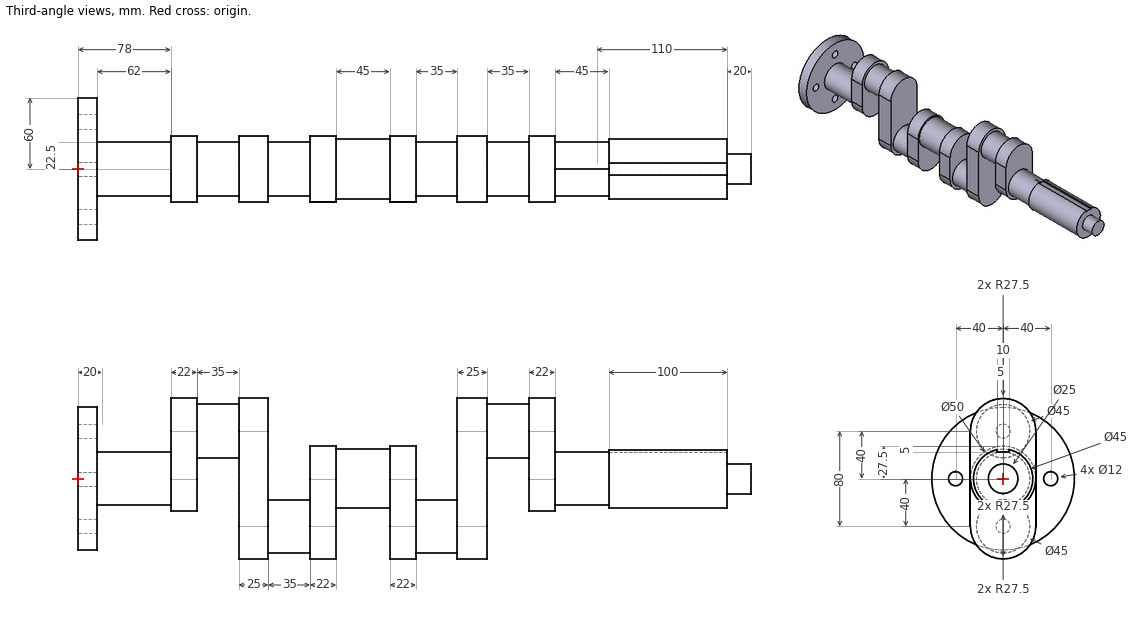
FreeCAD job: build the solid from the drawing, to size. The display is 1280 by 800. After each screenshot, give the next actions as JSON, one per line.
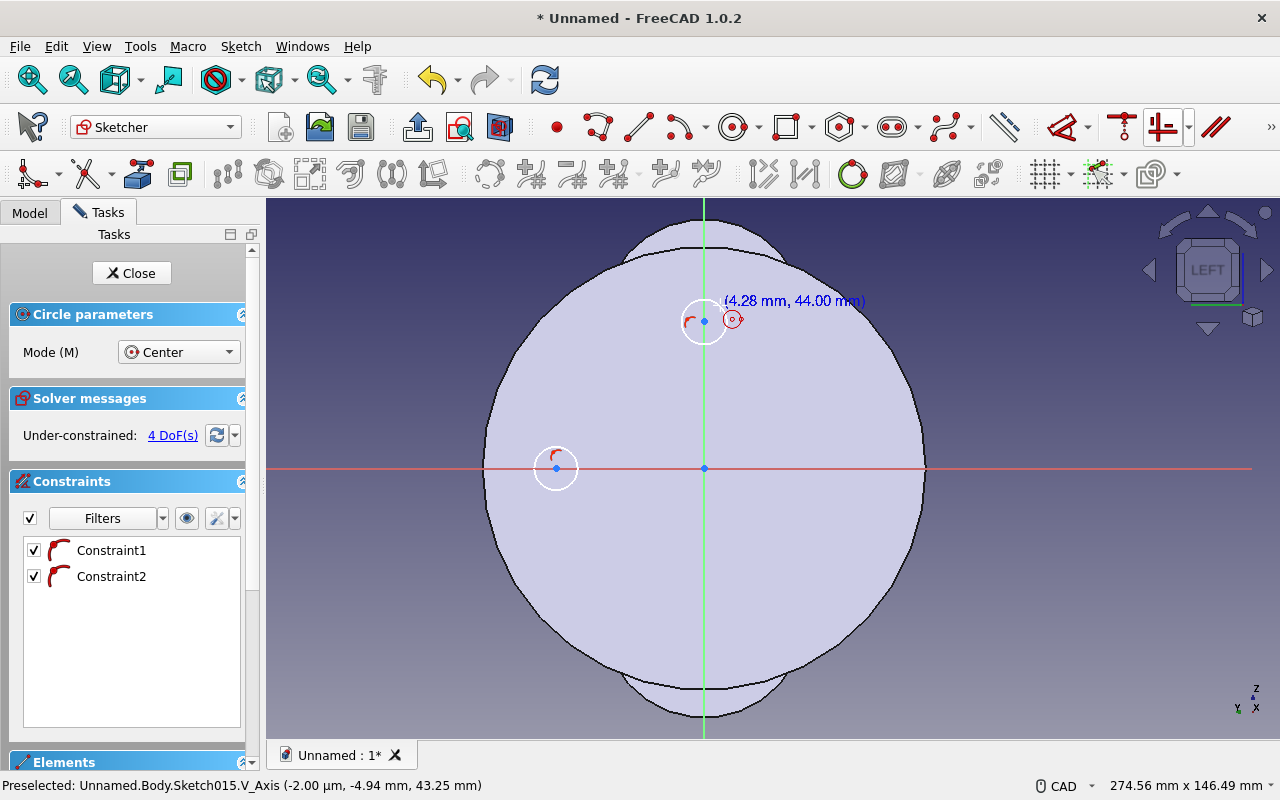
{"action": "left_click", "coordinate": [852, 468]}
{"action": "left_click", "coordinate": [868, 453]}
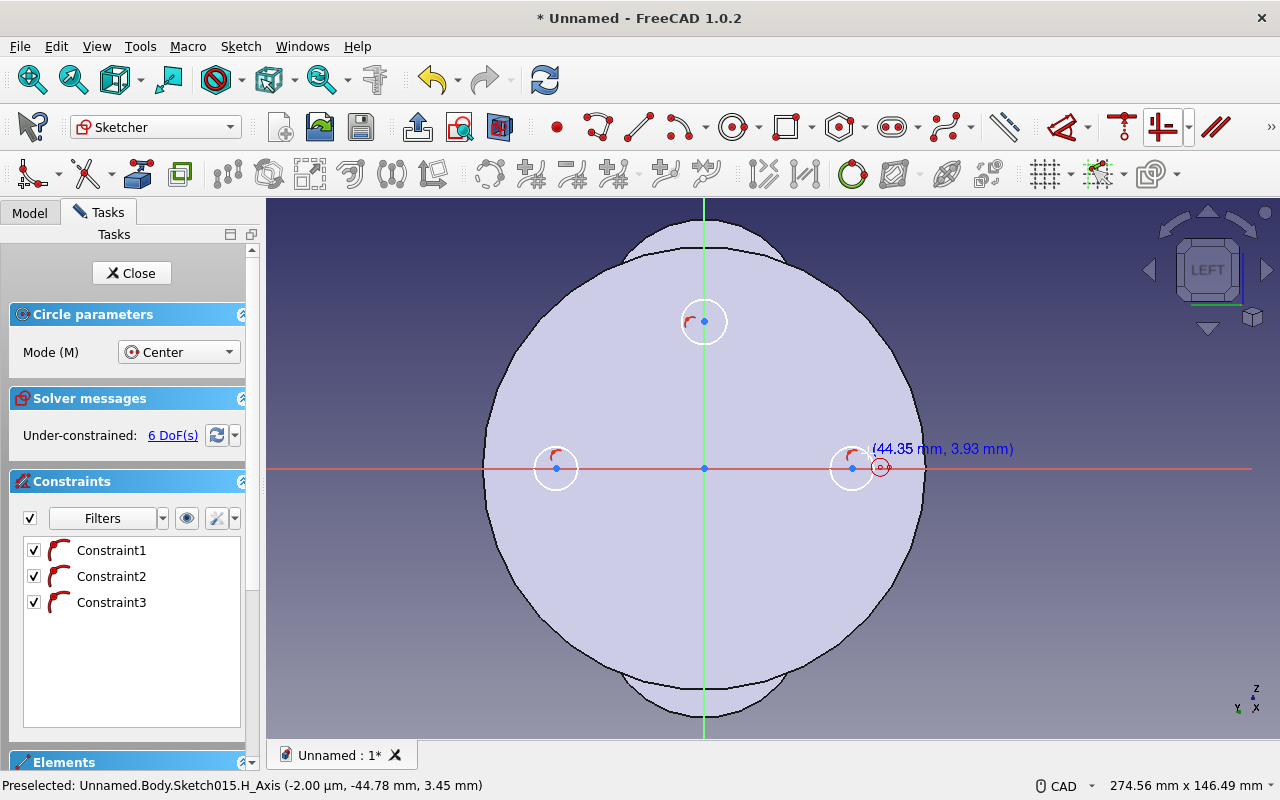
{"action": "left_click", "coordinate": [704, 616]}
{"action": "left_click", "coordinate": [720, 601]}
{"action": "key", "text": "Escape"}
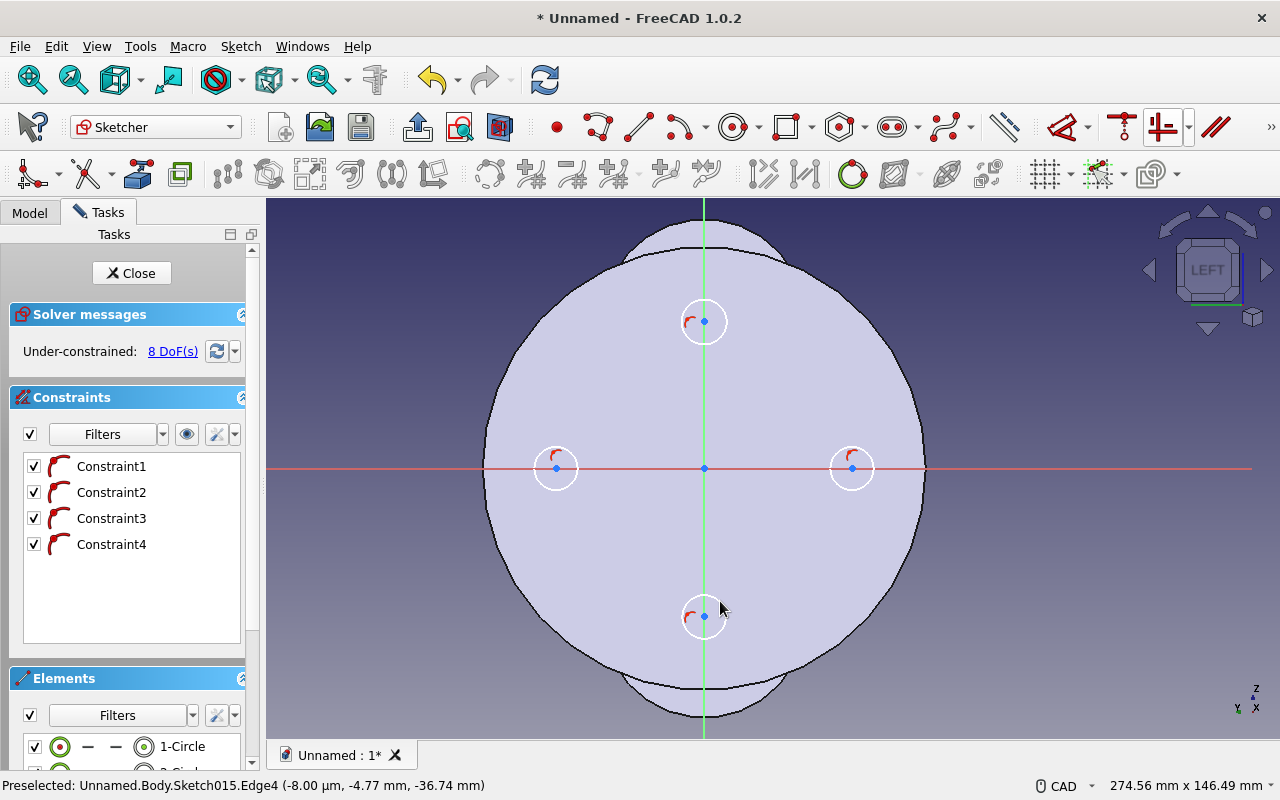
{"action": "left_click", "coordinate": [571, 453]}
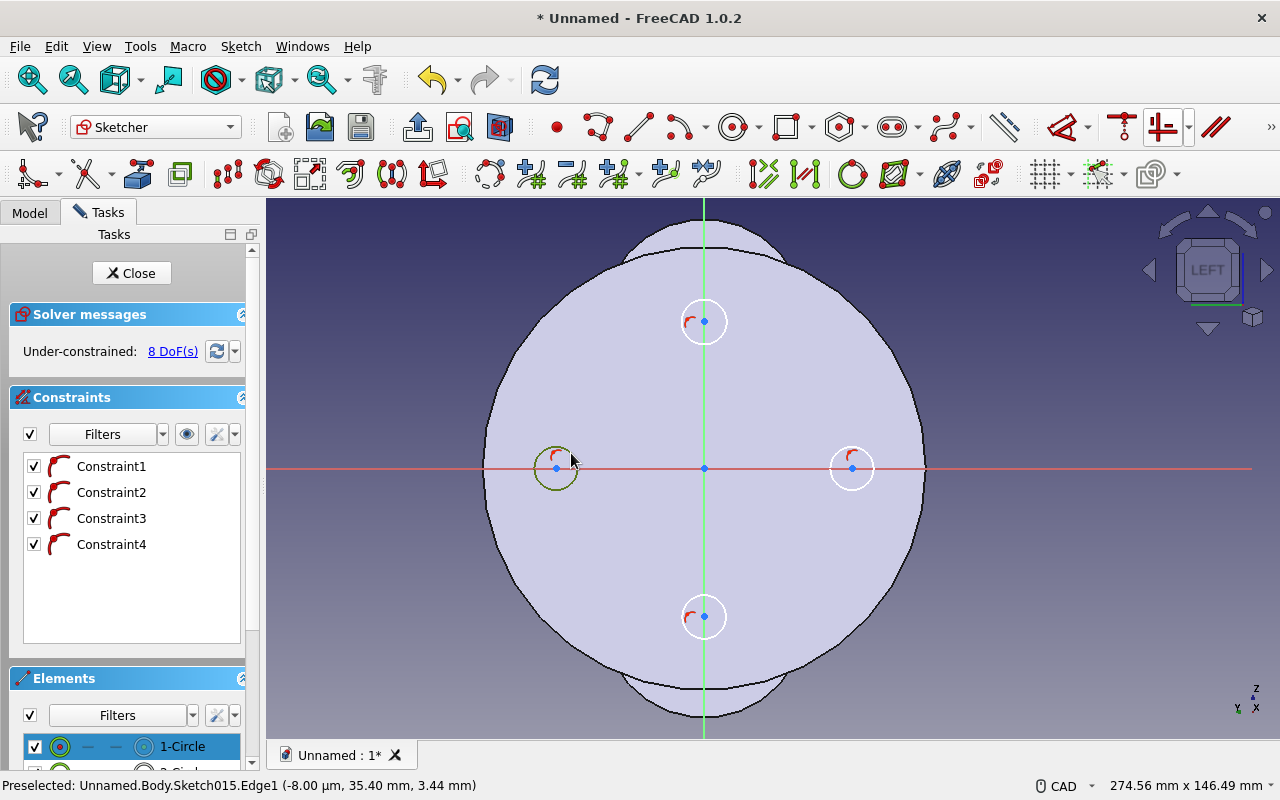
{"action": "left_click", "coordinate": [720, 306]}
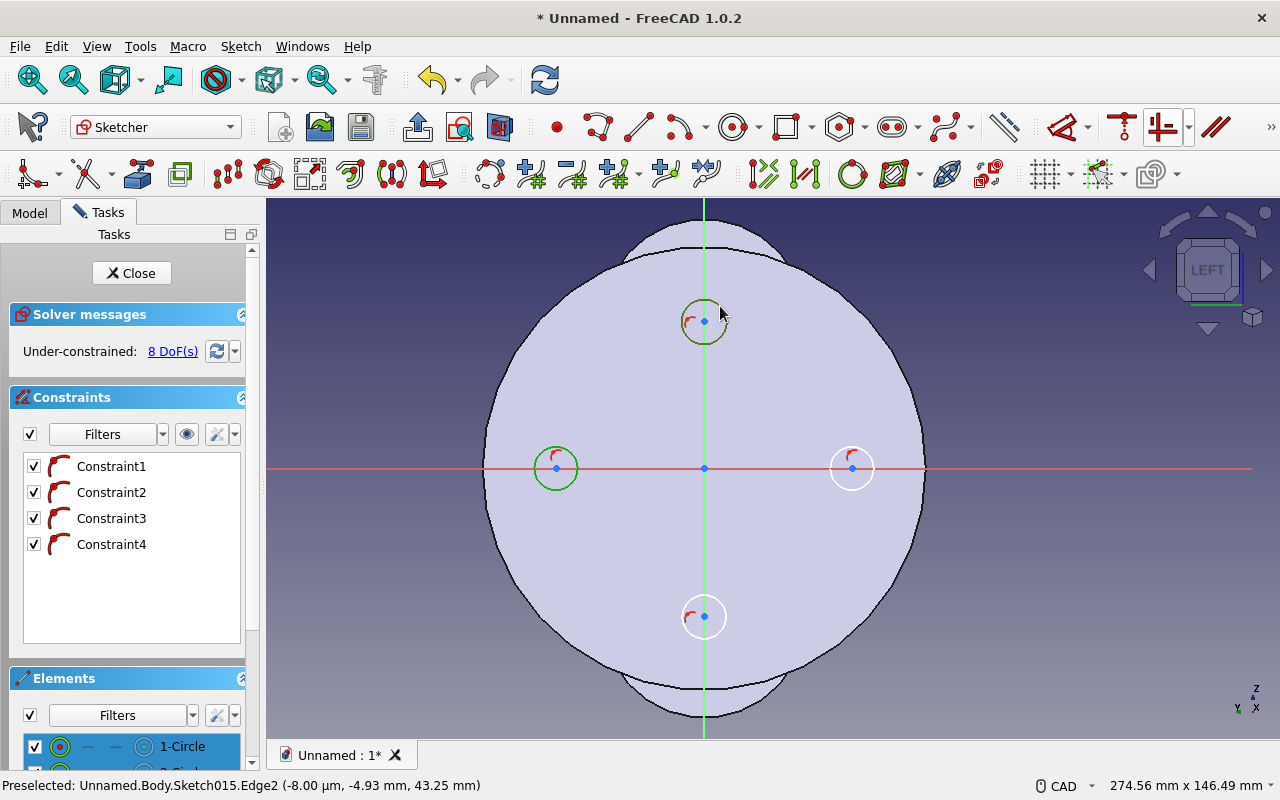
{"action": "left_click", "coordinate": [867, 453]}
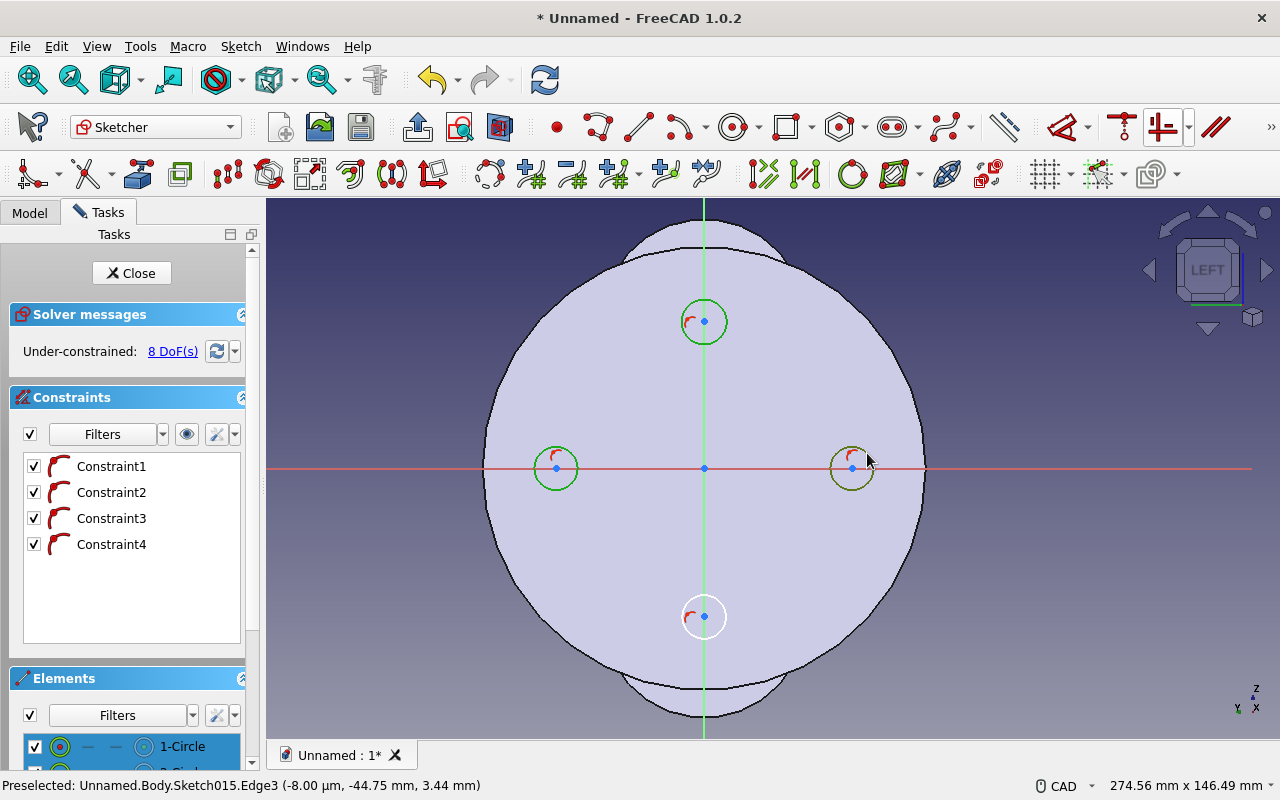
{"action": "left_click", "coordinate": [720, 602]}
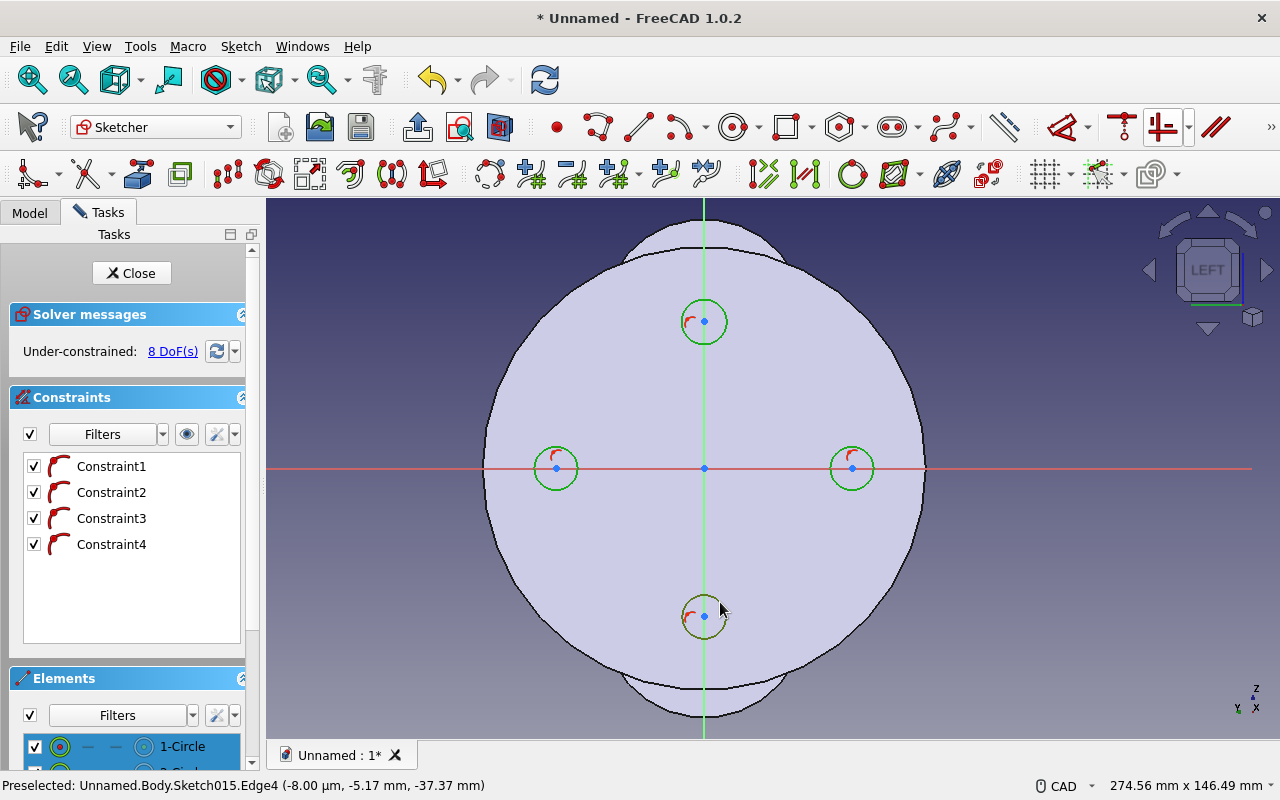
{"action": "key", "text": "e"}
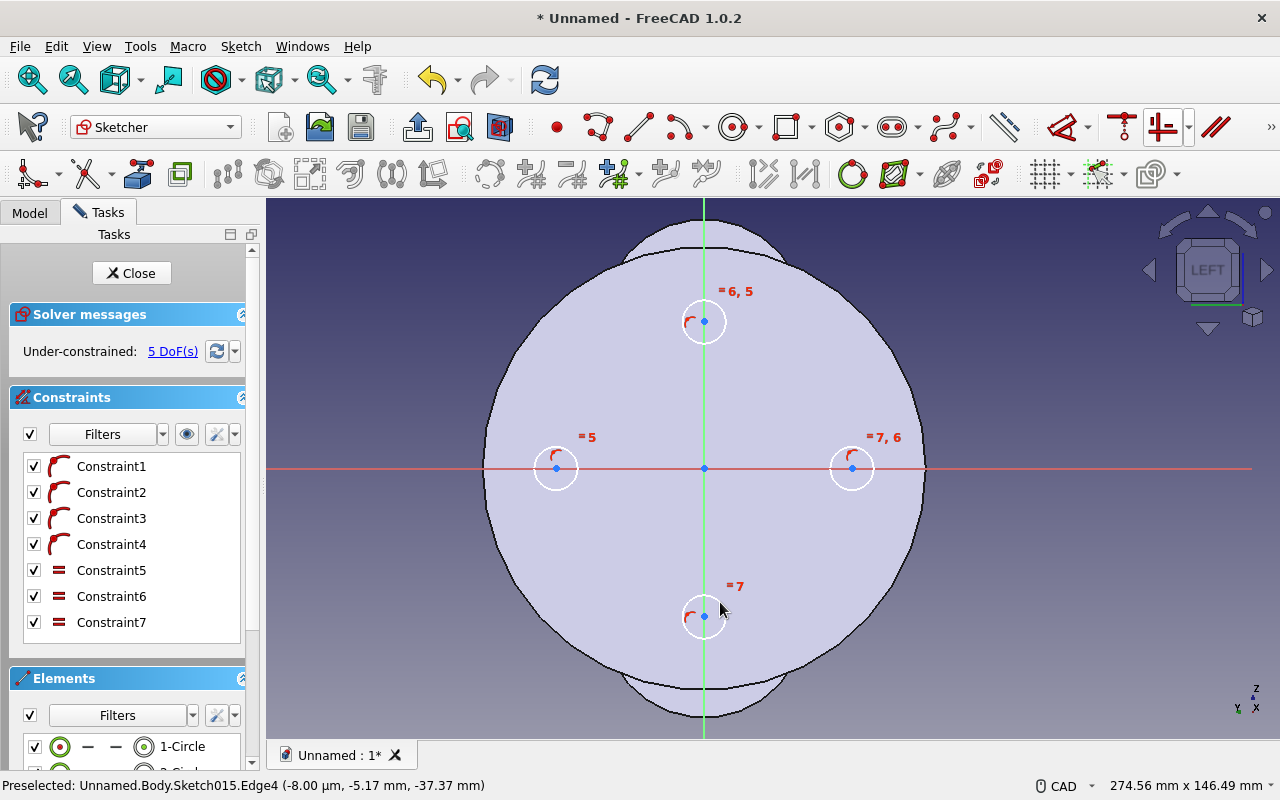
{"action": "left_click", "coordinate": [1062, 128]}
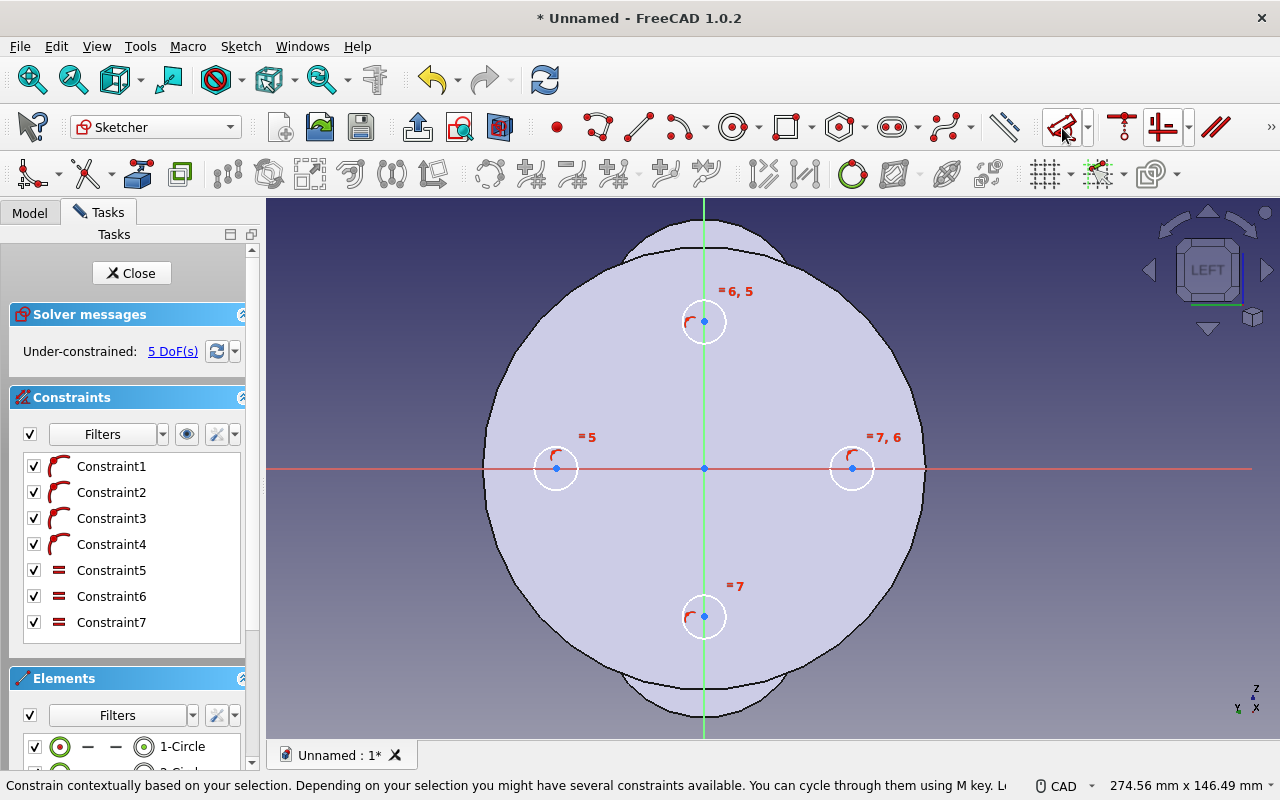
{"action": "left_click", "coordinate": [571, 453]}
{"action": "left_click", "coordinate": [593, 430]}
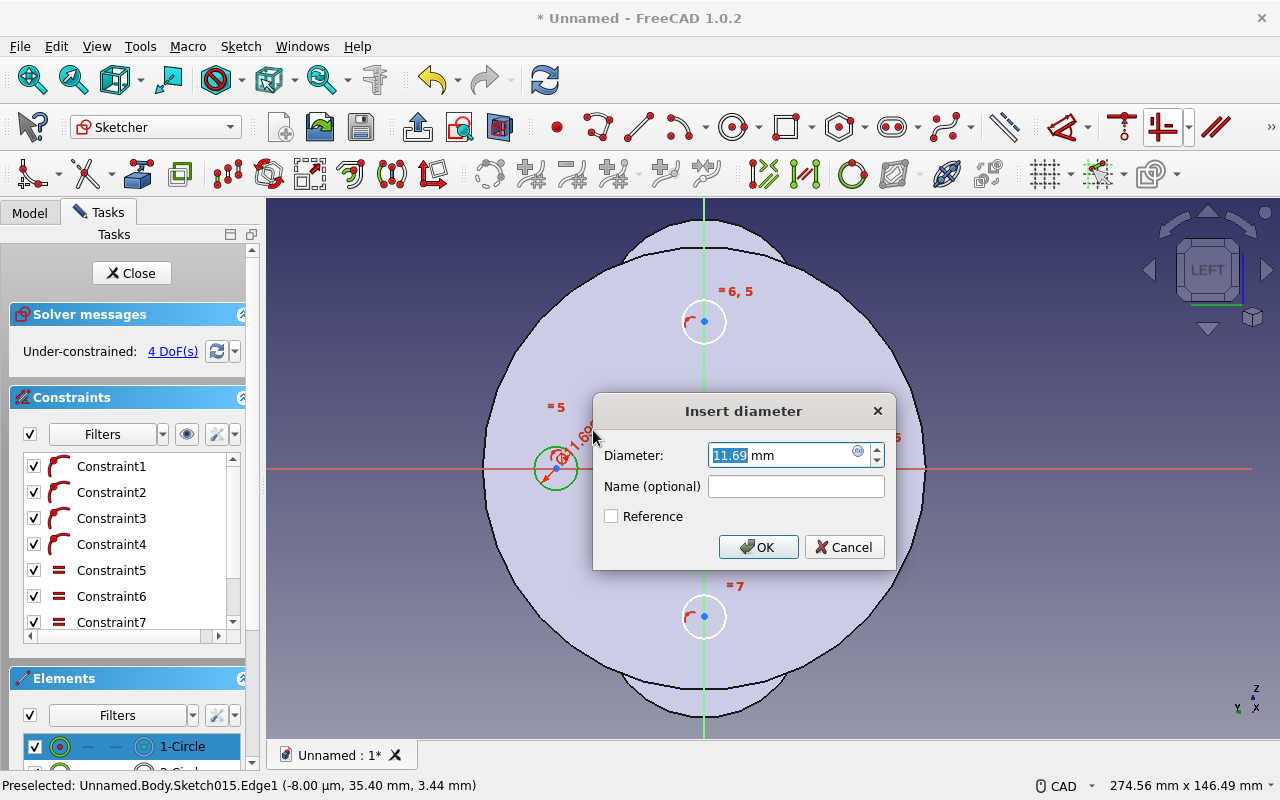
{"action": "type", "text": "12"}
{"action": "key", "text": "Return"}